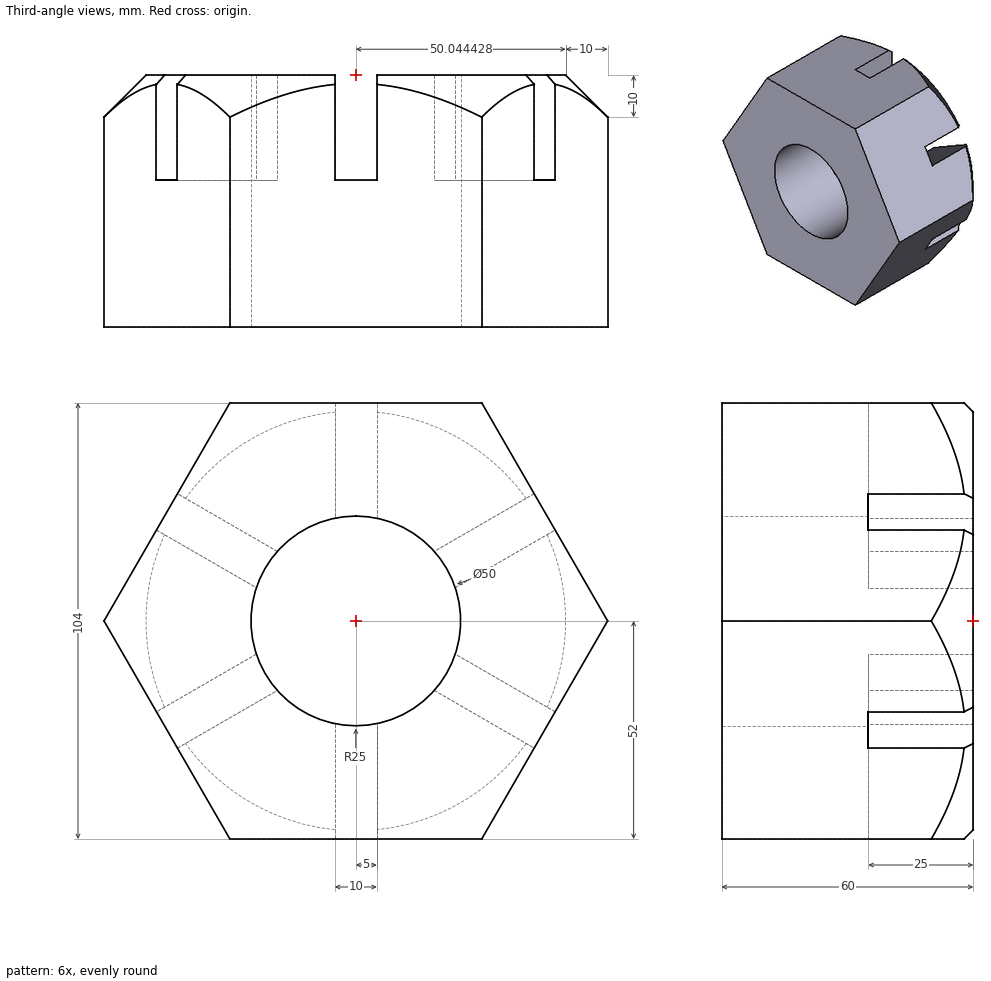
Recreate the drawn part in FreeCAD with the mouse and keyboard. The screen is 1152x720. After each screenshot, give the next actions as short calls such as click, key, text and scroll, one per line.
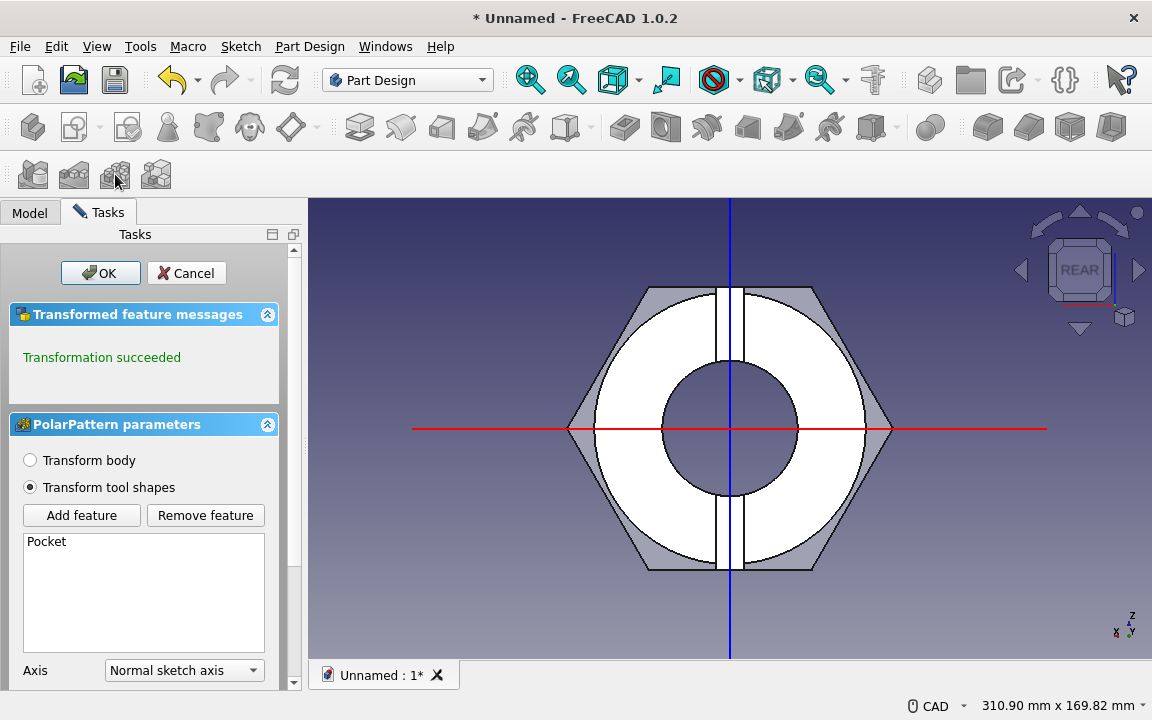
click(185, 670)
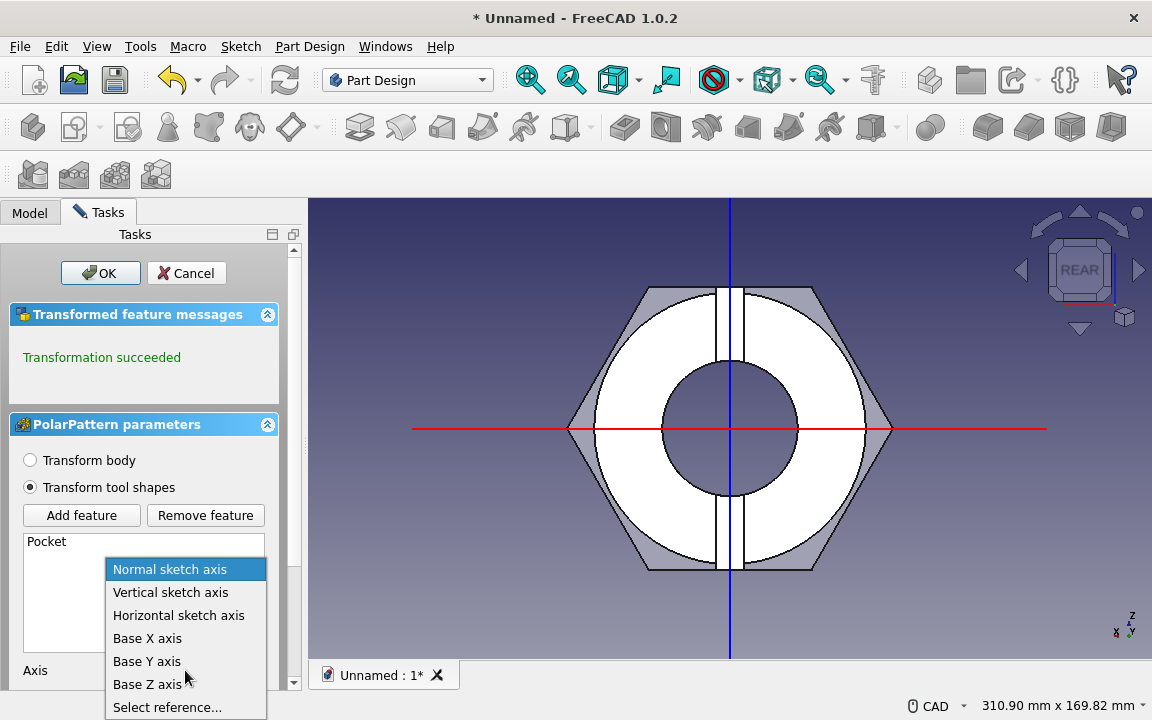
click(184, 662)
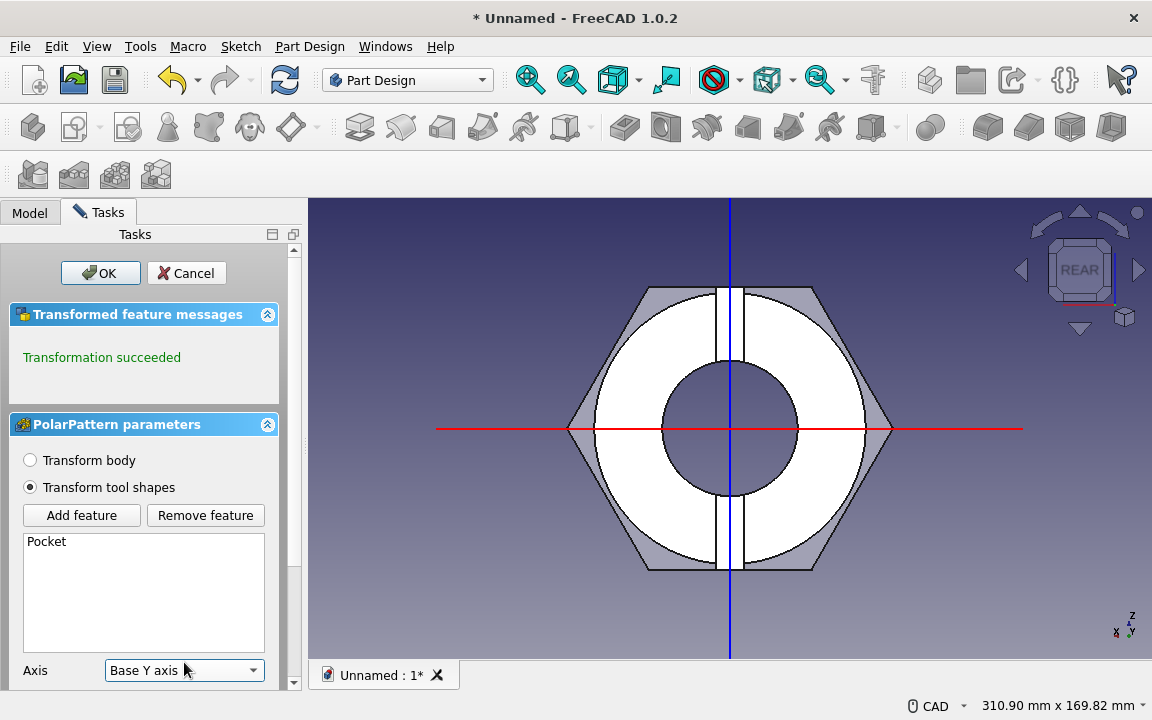
scroll(294, 467, down, 3)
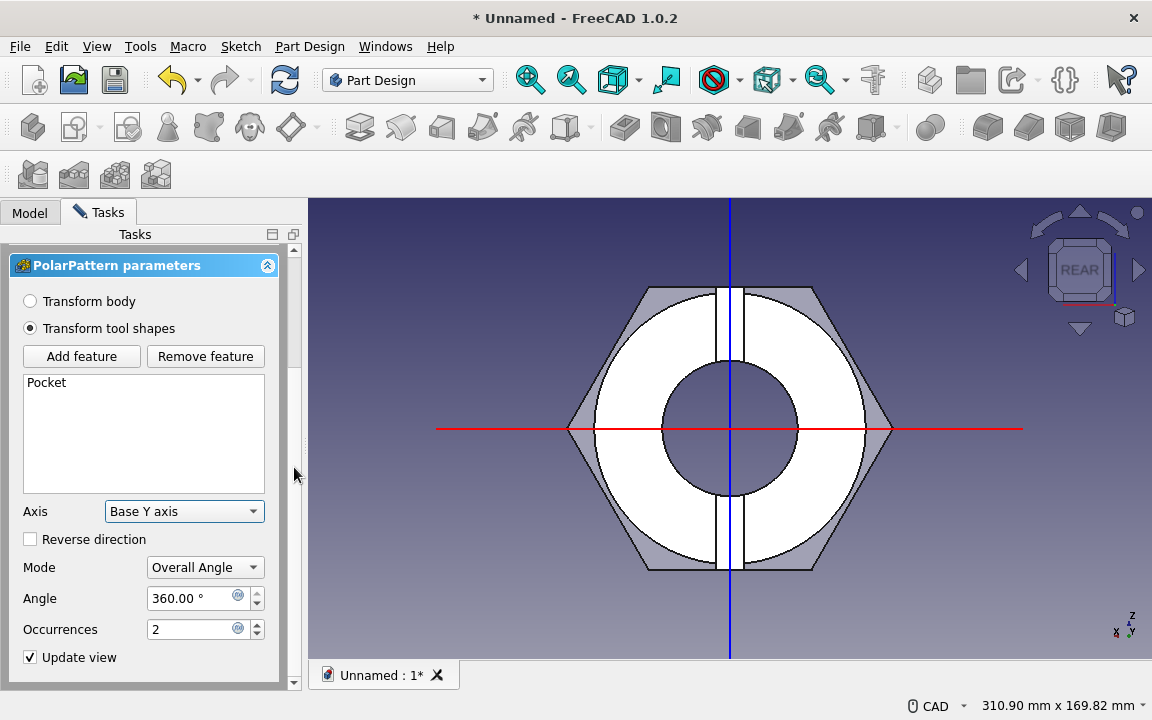
triple_click(199, 630)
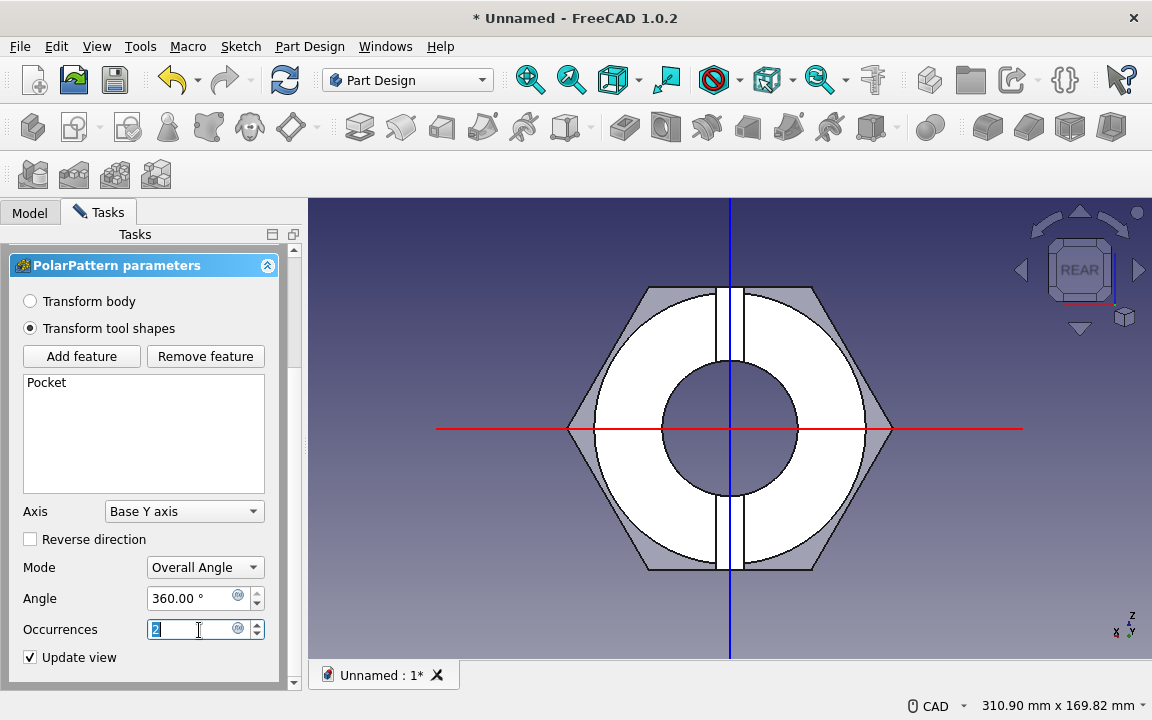
text(6)
key(Tab)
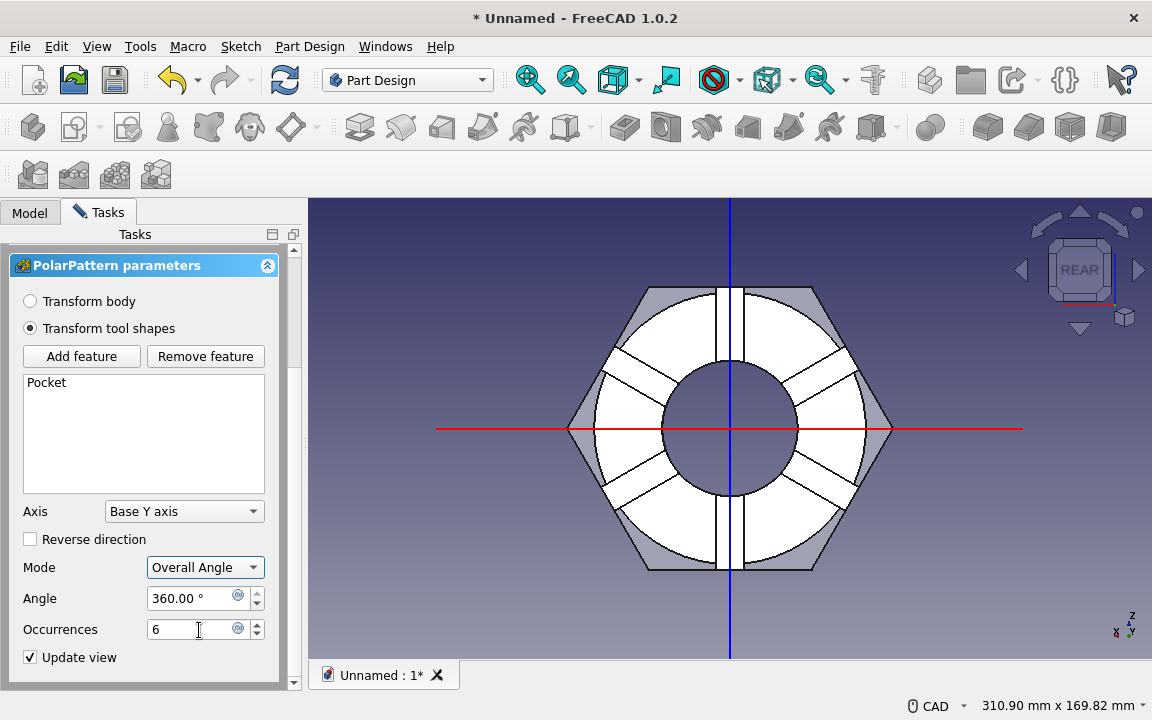
scroll(294, 467, up, 4)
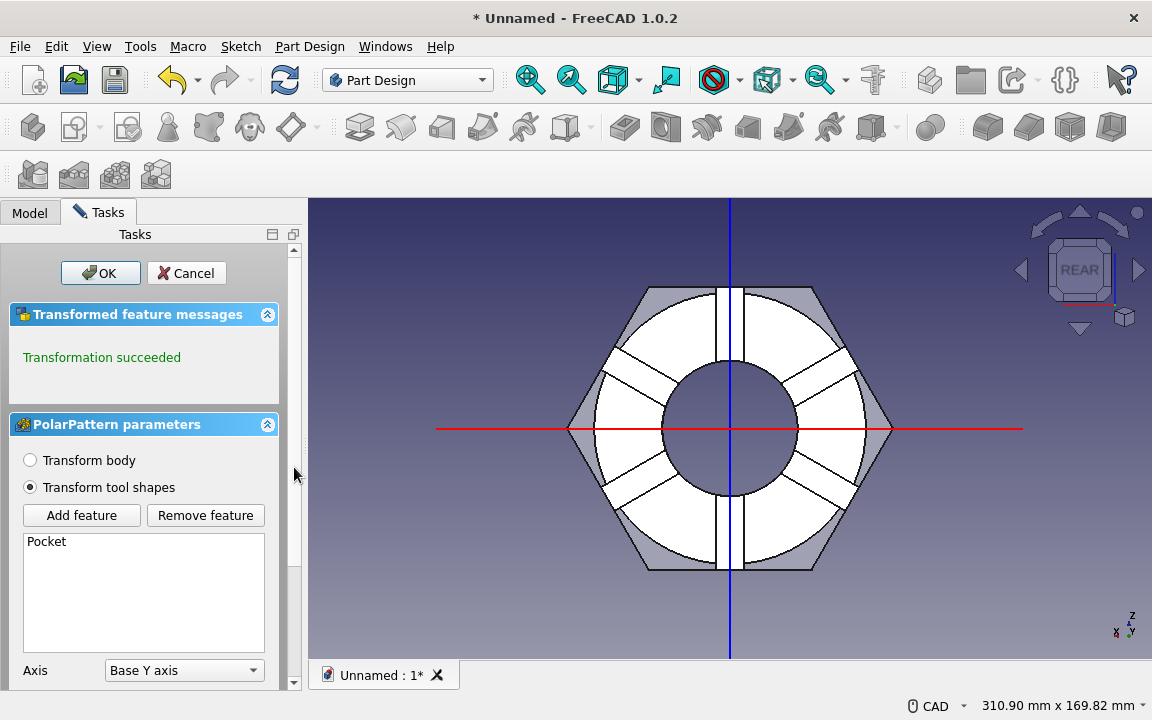
click(101, 273)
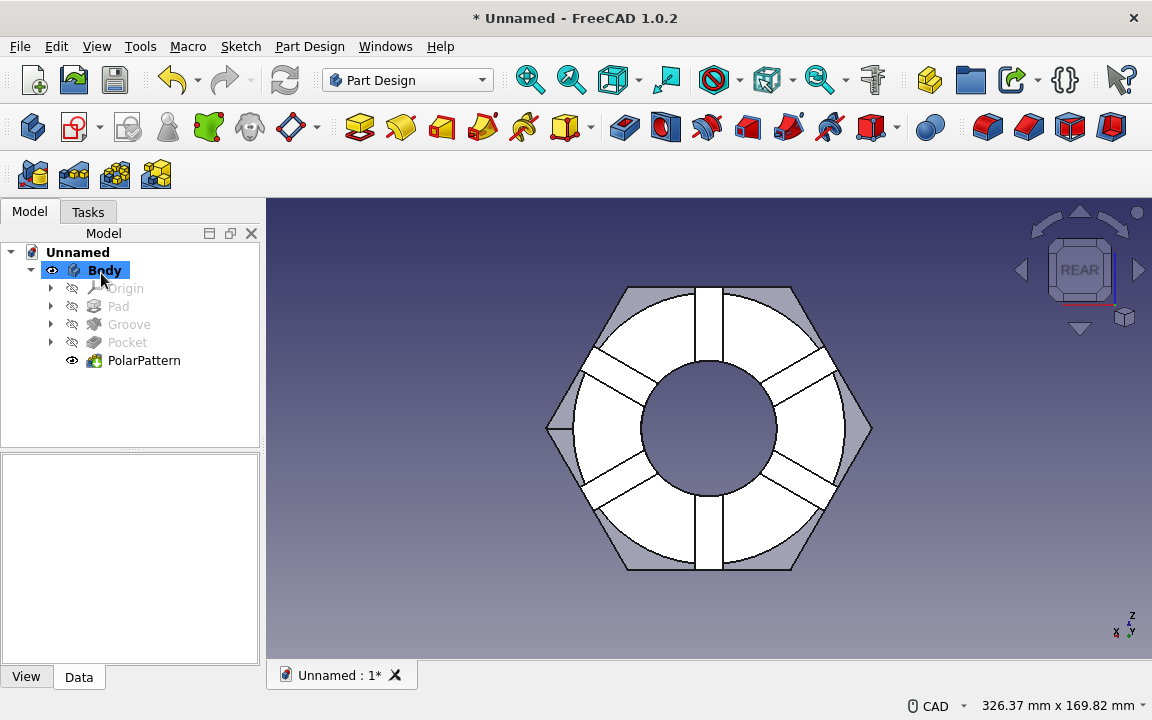
key(0)